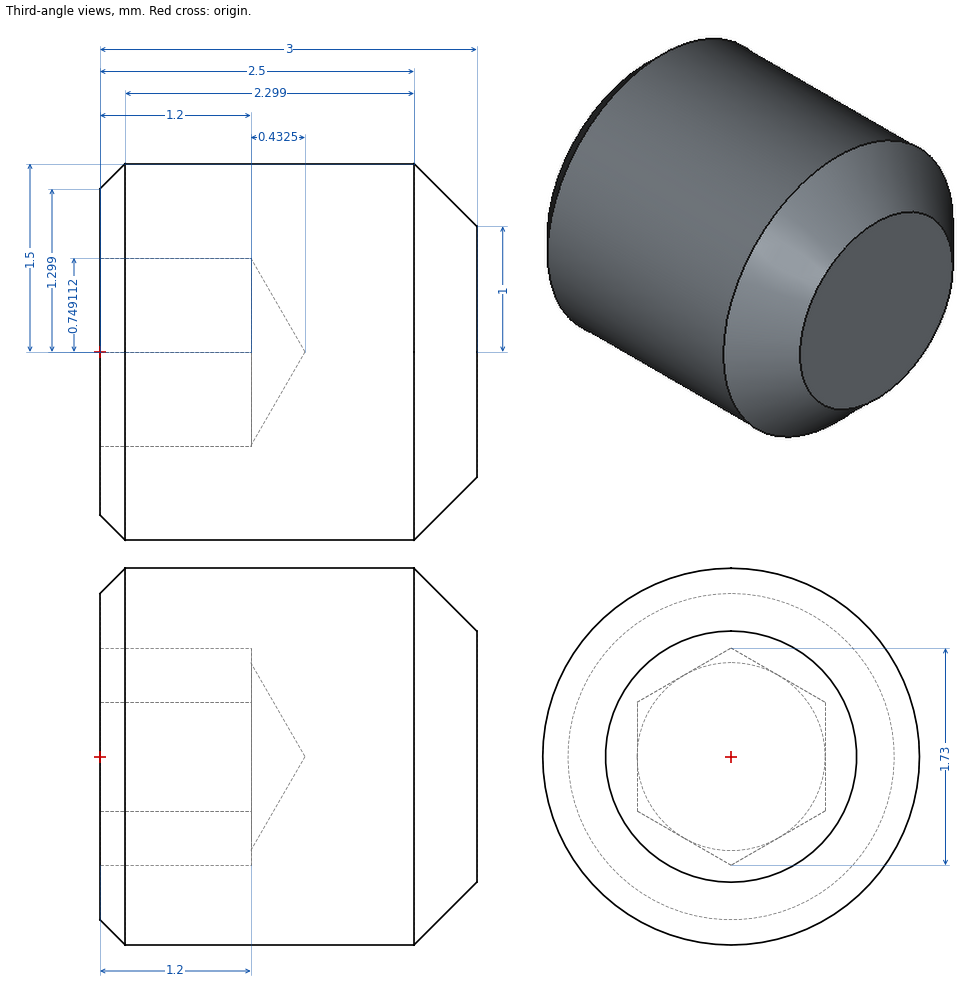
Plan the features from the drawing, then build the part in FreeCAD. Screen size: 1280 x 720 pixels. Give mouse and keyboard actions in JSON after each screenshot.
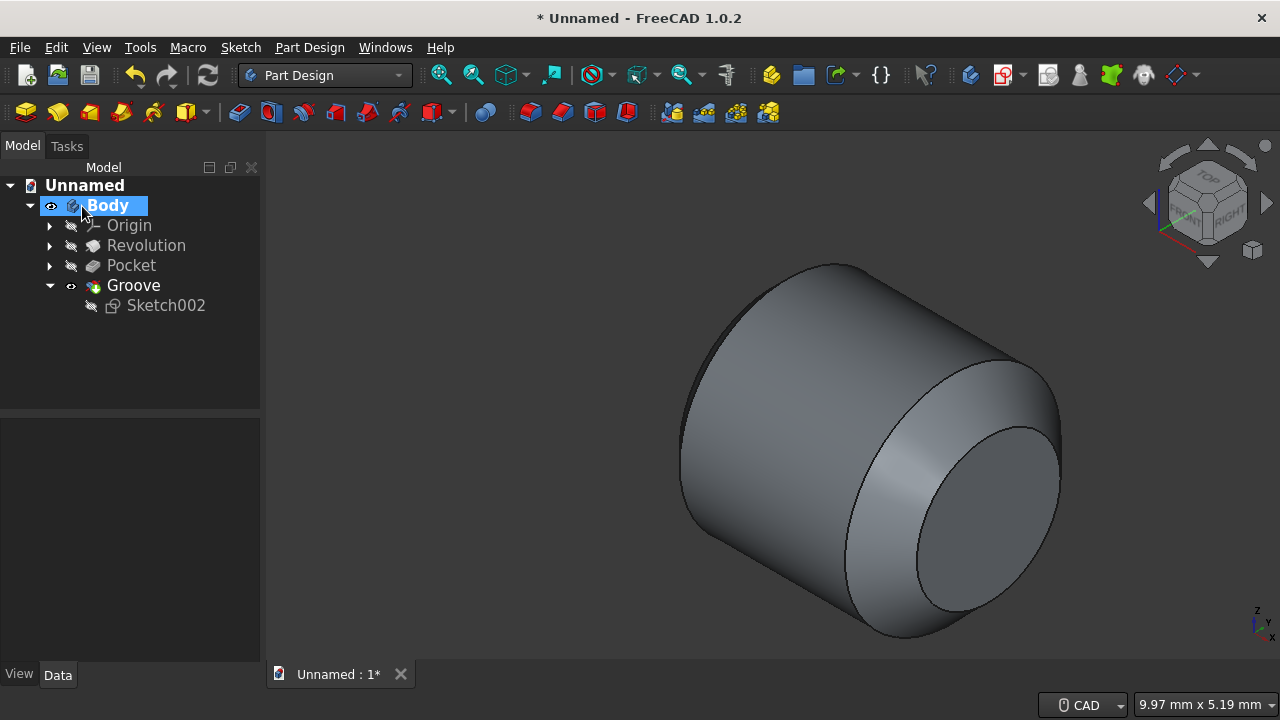
{"action": "left_click", "coordinate": [442, 76]}